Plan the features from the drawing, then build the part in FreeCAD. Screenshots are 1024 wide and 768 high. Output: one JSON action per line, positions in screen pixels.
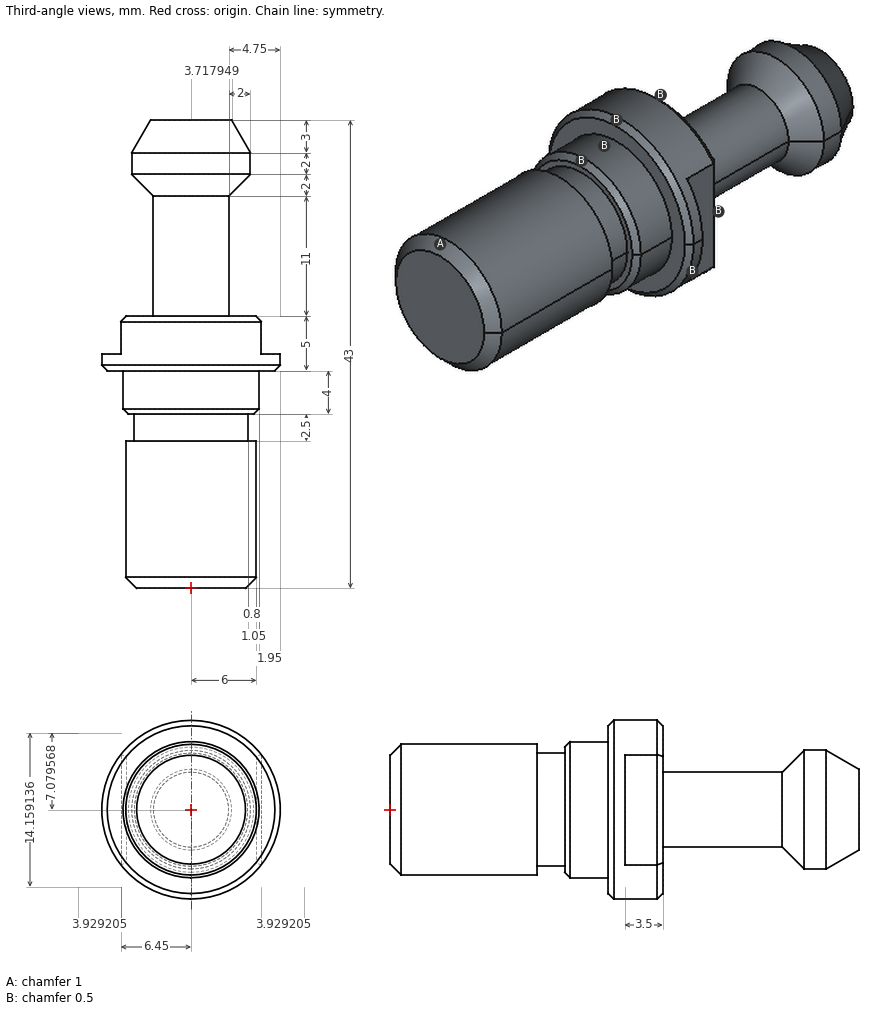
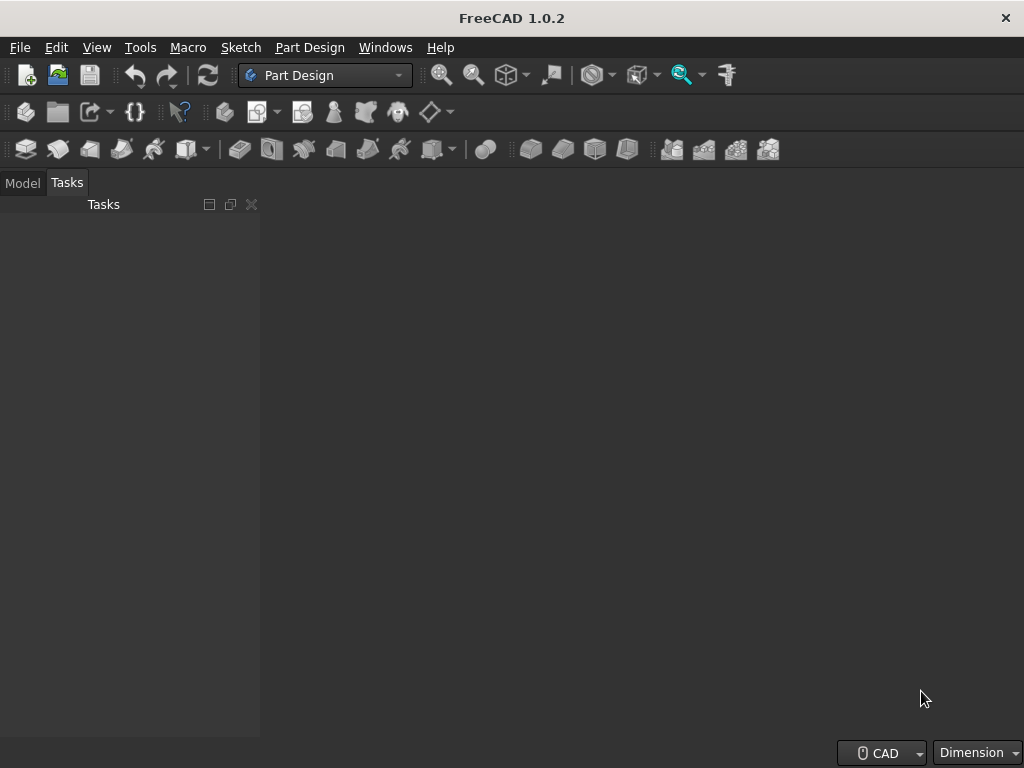
{"action": "left_click", "coordinate": [26, 76]}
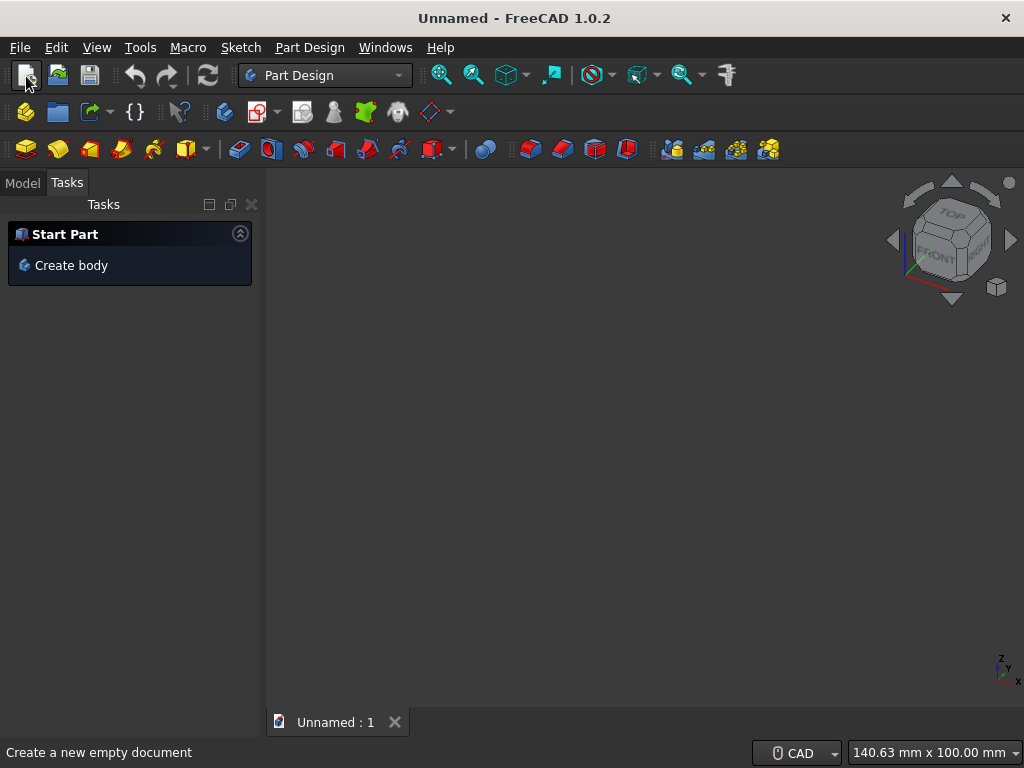
{"action": "left_click", "coordinate": [258, 112]}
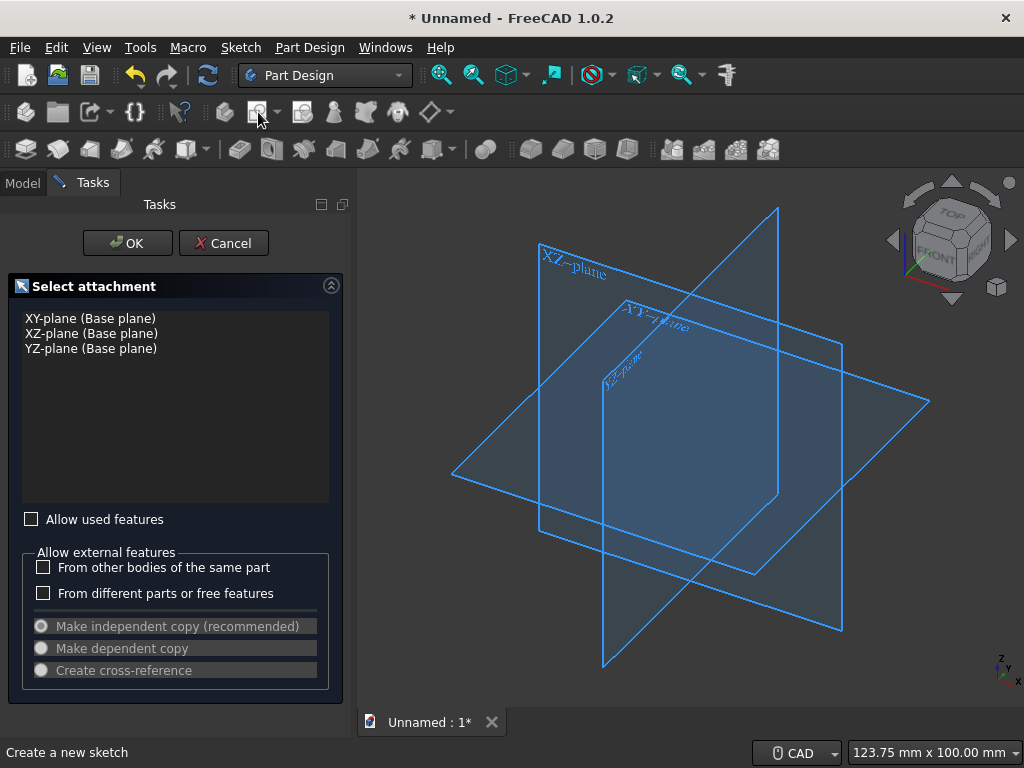
{"action": "left_click", "coordinate": [82, 318]}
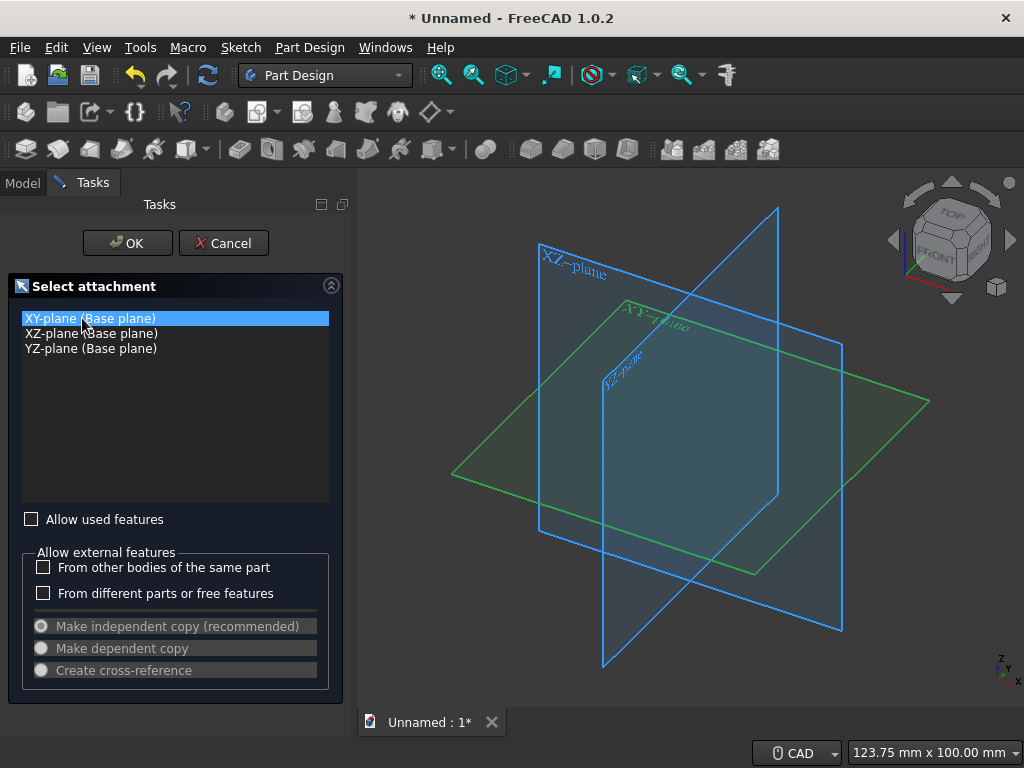
{"action": "left_click", "coordinate": [128, 243]}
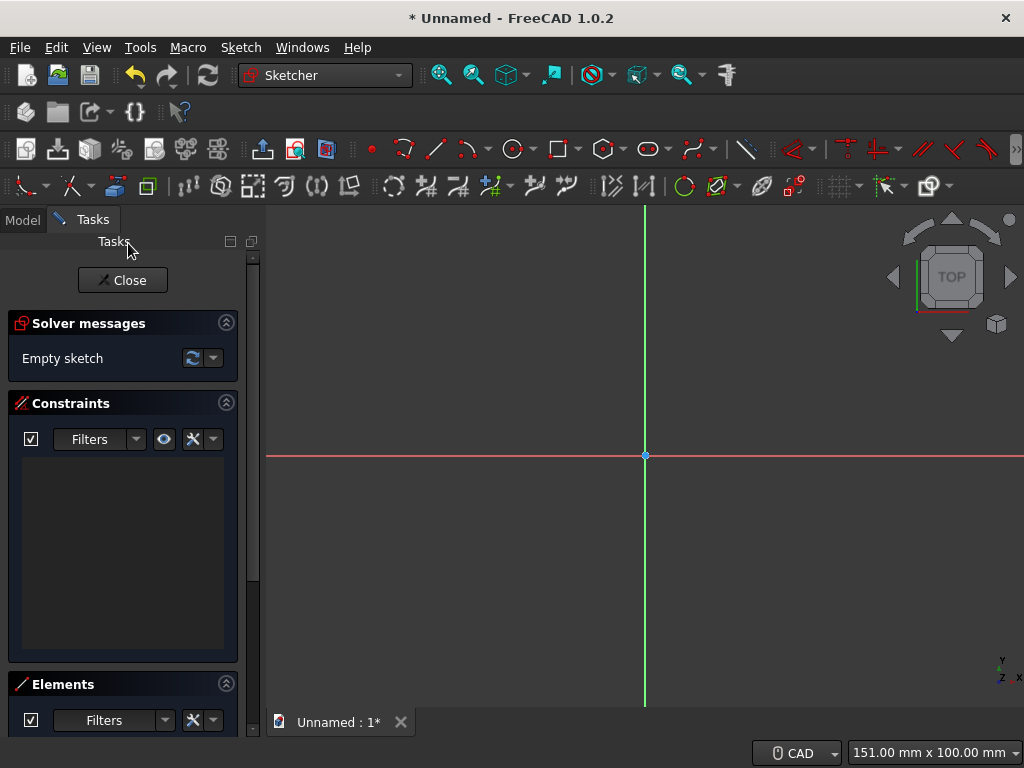
{"action": "scroll", "coordinate": [294, 679], "scroll_direction": "down", "scroll_amount": 1}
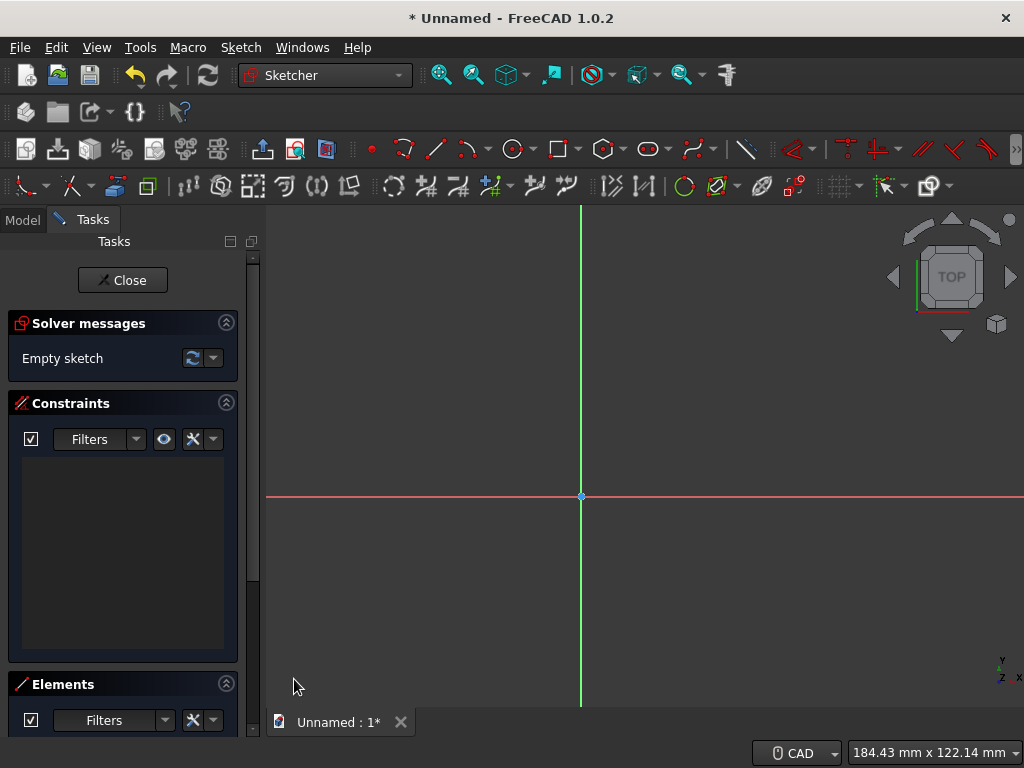
{"action": "scroll", "coordinate": [625, 350], "scroll_direction": "up", "scroll_amount": 3}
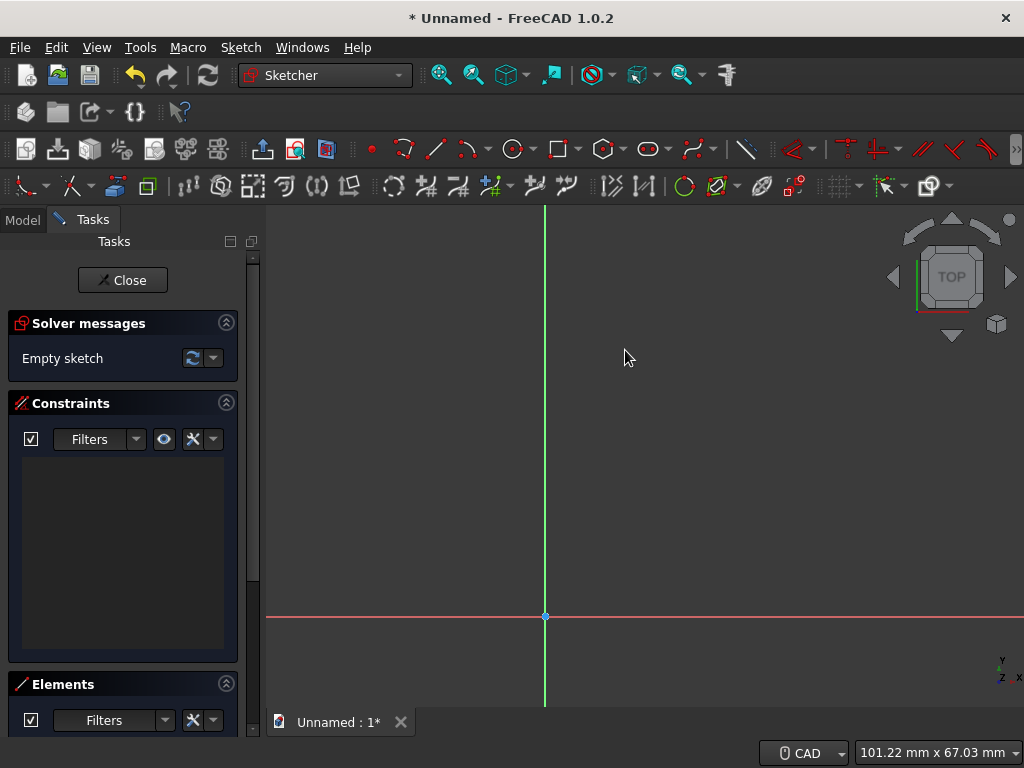
{"action": "left_click", "coordinate": [404, 150]}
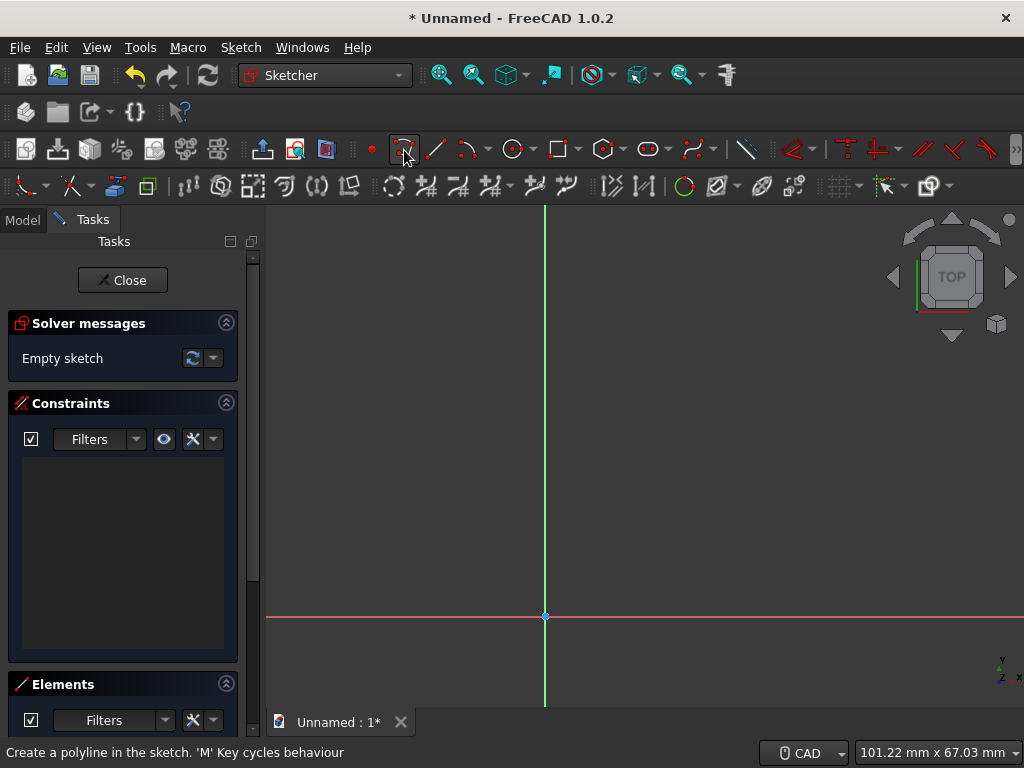
{"action": "left_click", "coordinate": [545, 617]}
{"action": "left_click", "coordinate": [590, 608]}
{"action": "left_click", "coordinate": [590, 516]}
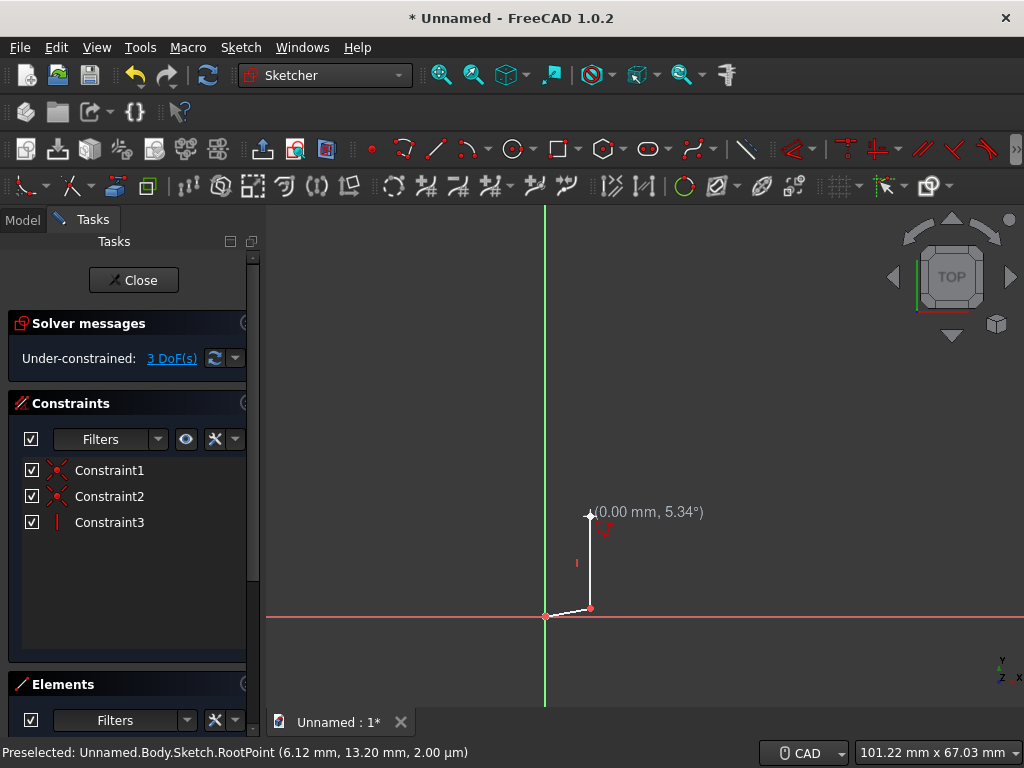
{"action": "scroll", "coordinate": [584, 516], "scroll_direction": "up", "scroll_amount": 5}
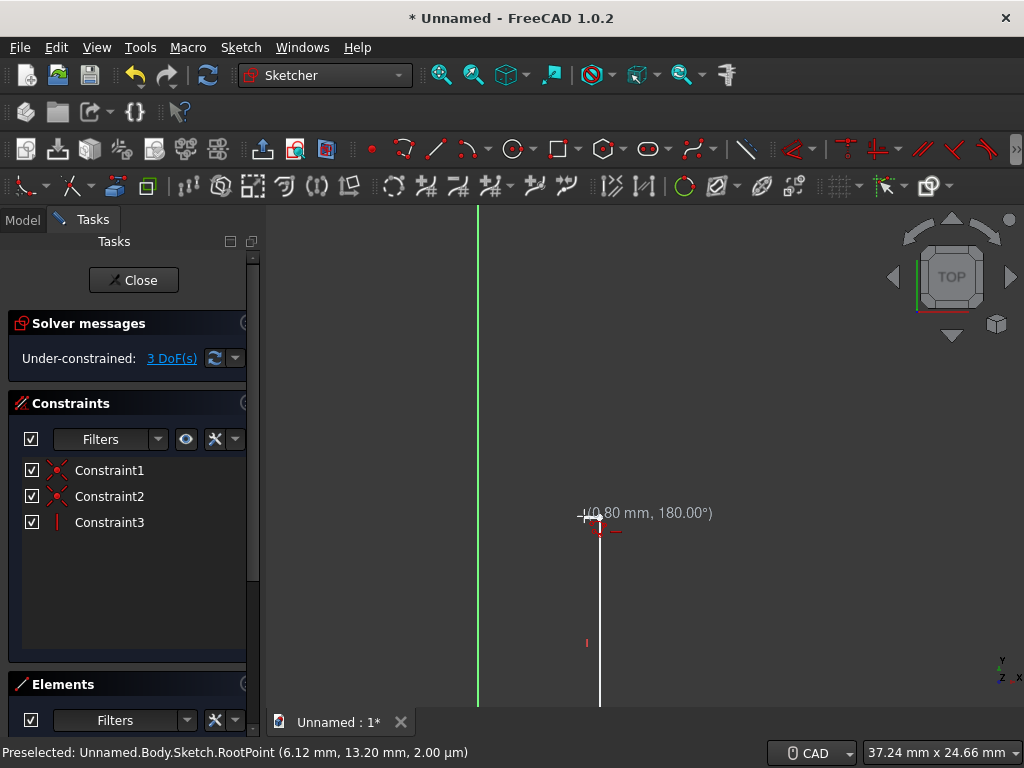
{"action": "left_click", "coordinate": [583, 515]}
{"action": "left_click", "coordinate": [583, 463]}
{"action": "left_click", "coordinate": [605, 463]}
{"action": "left_click", "coordinate": [605, 382]}
{"action": "left_click", "coordinate": [645, 382]}
{"action": "left_click", "coordinate": [645, 280]}
{"action": "left_click", "coordinate": [548, 280]}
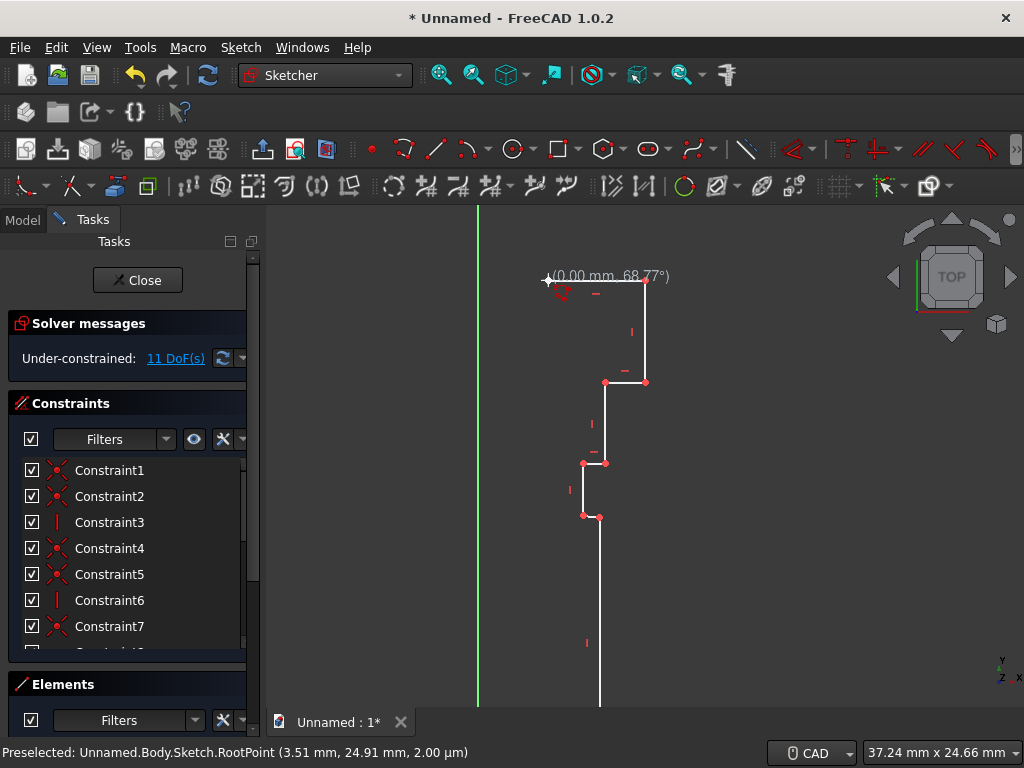
{"action": "scroll", "coordinate": [585, 517], "scroll_direction": "down", "scroll_amount": 5}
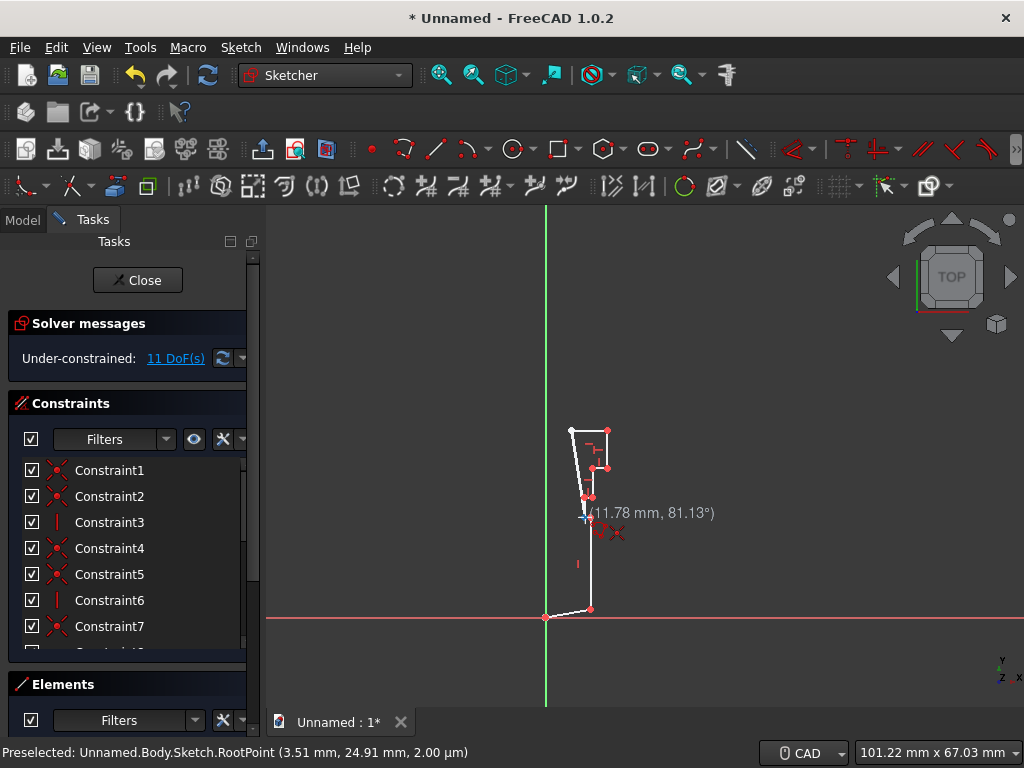
{"action": "left_click", "coordinate": [572, 348]}
{"action": "left_click", "coordinate": [587, 333]}
{"action": "left_click", "coordinate": [587, 318]}
{"action": "left_click", "coordinate": [574, 295]}
{"action": "left_click", "coordinate": [555, 295]}
{"action": "left_click", "coordinate": [546, 618]}
{"action": "key", "text": "Escape"}
{"action": "key", "text": "Escape"}